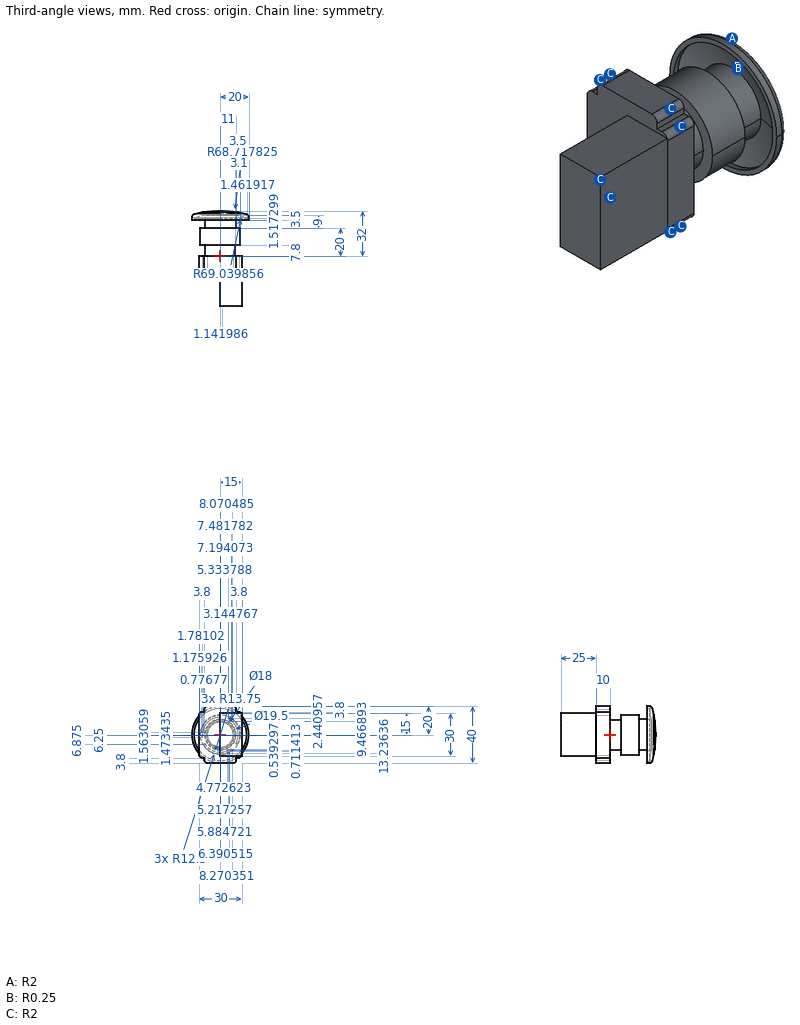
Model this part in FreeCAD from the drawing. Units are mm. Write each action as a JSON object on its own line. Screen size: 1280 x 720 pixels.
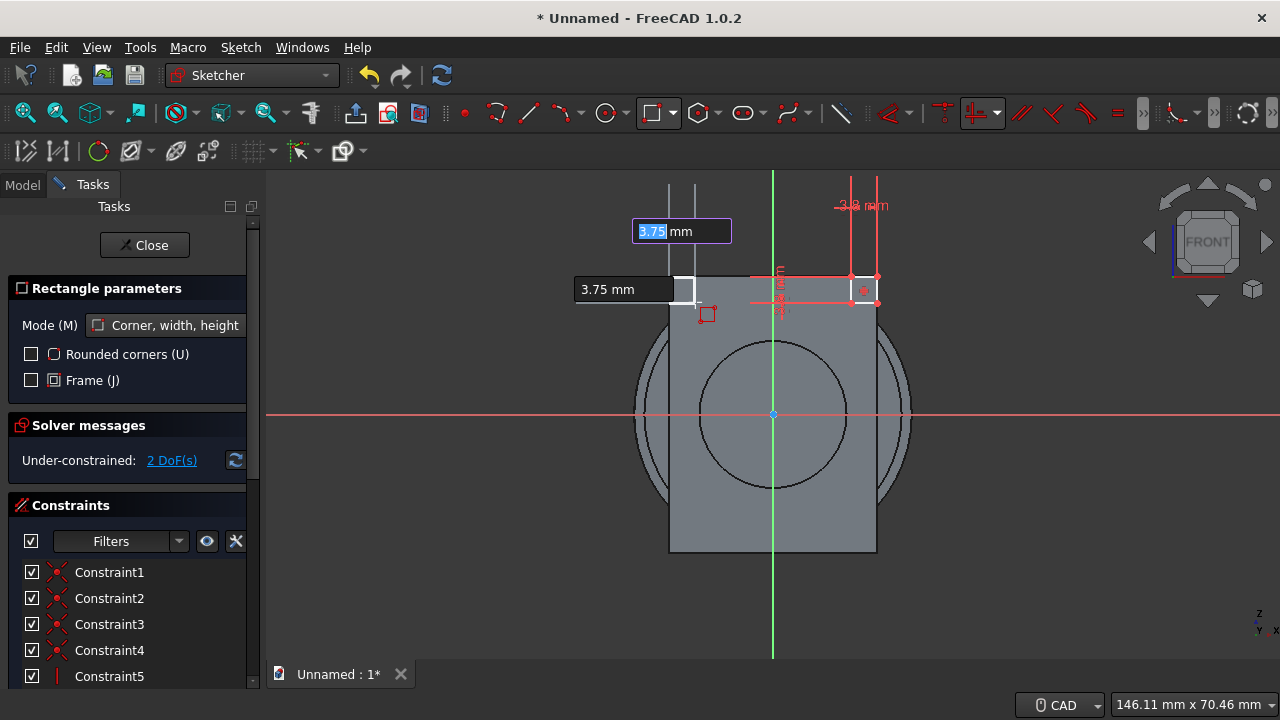
{"action": "type", "text": "3.8"}
{"action": "key", "text": "Tab"}
{"action": "type", "text": "3.8"}
{"action": "key", "text": "Return"}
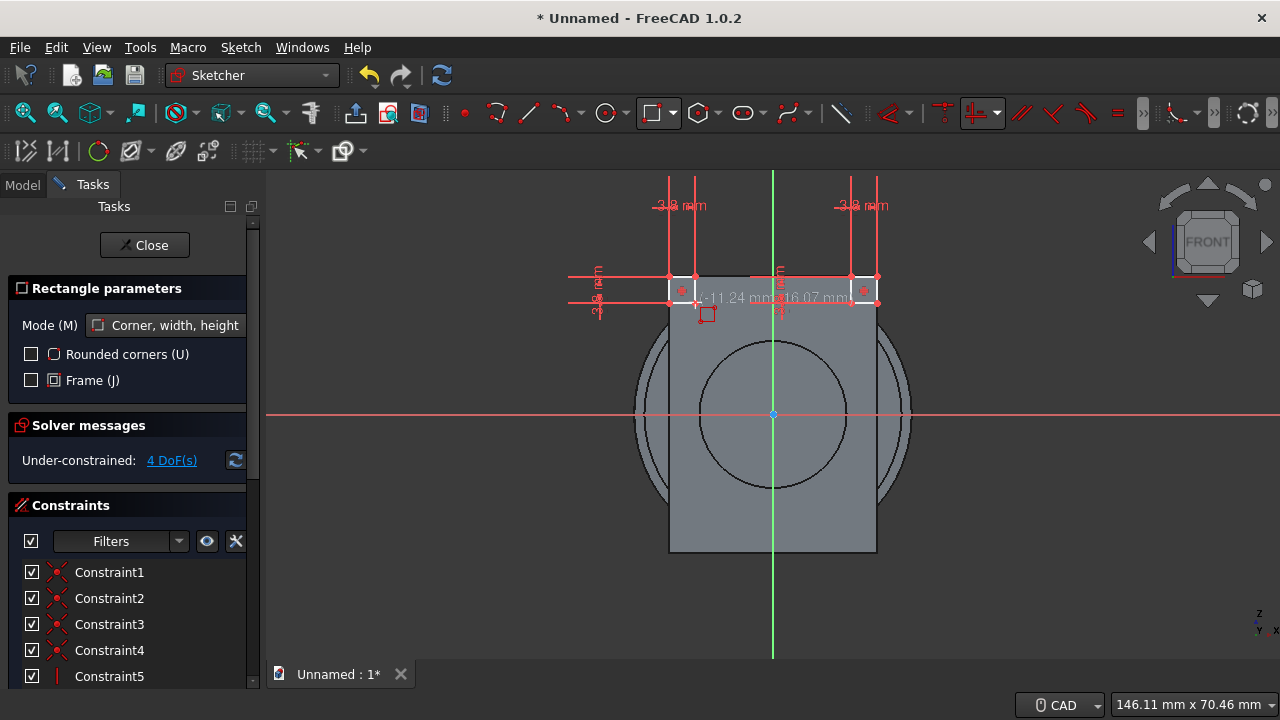
{"action": "left_click", "coordinate": [669, 527]}
{"action": "mouse_move", "coordinate": [695, 553]}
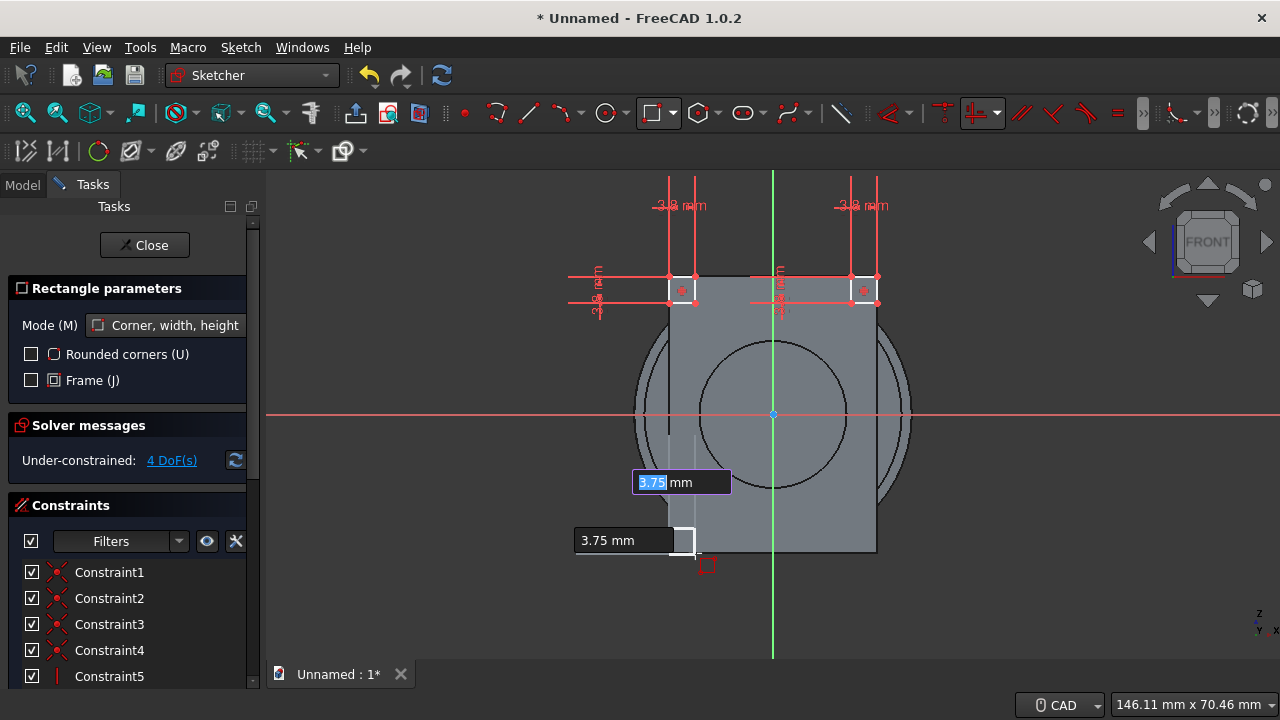
{"action": "type", "text": "3.8"}
{"action": "key", "text": "Tab"}
{"action": "type", "text": "3.8"}
{"action": "key", "text": "Return"}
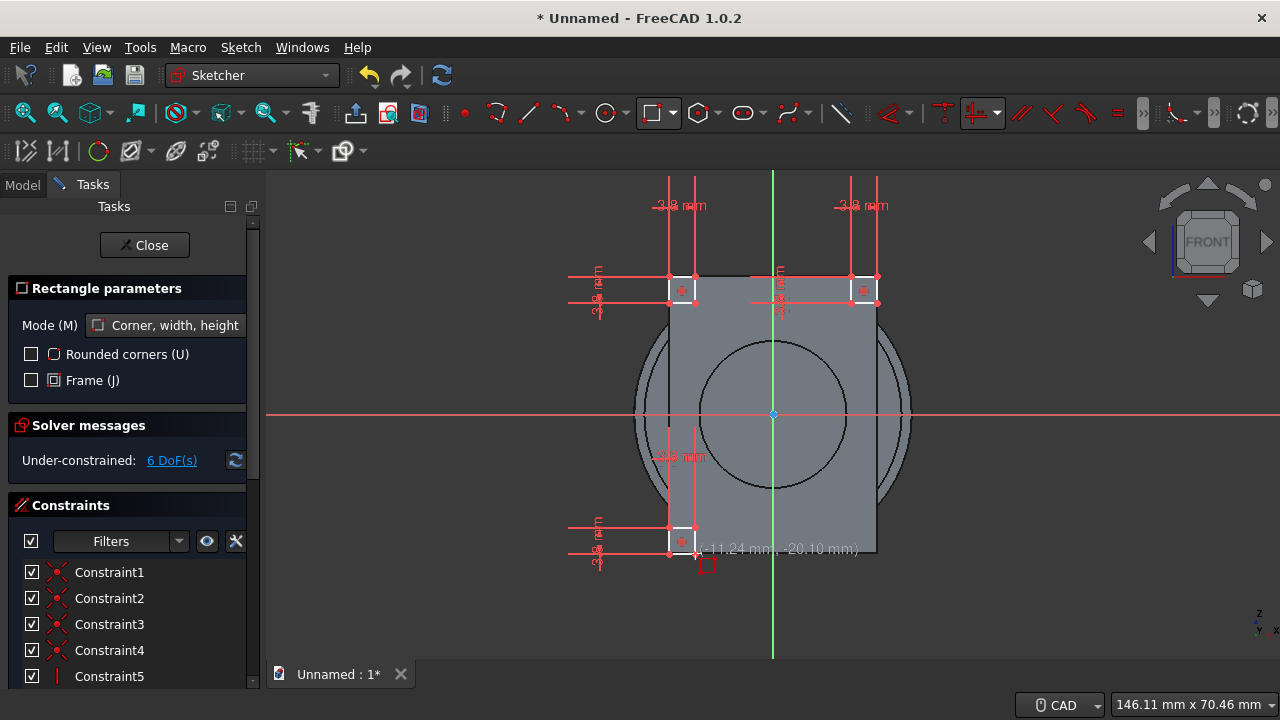
{"action": "left_click", "coordinate": [851, 527]}
{"action": "mouse_move", "coordinate": [877, 553]}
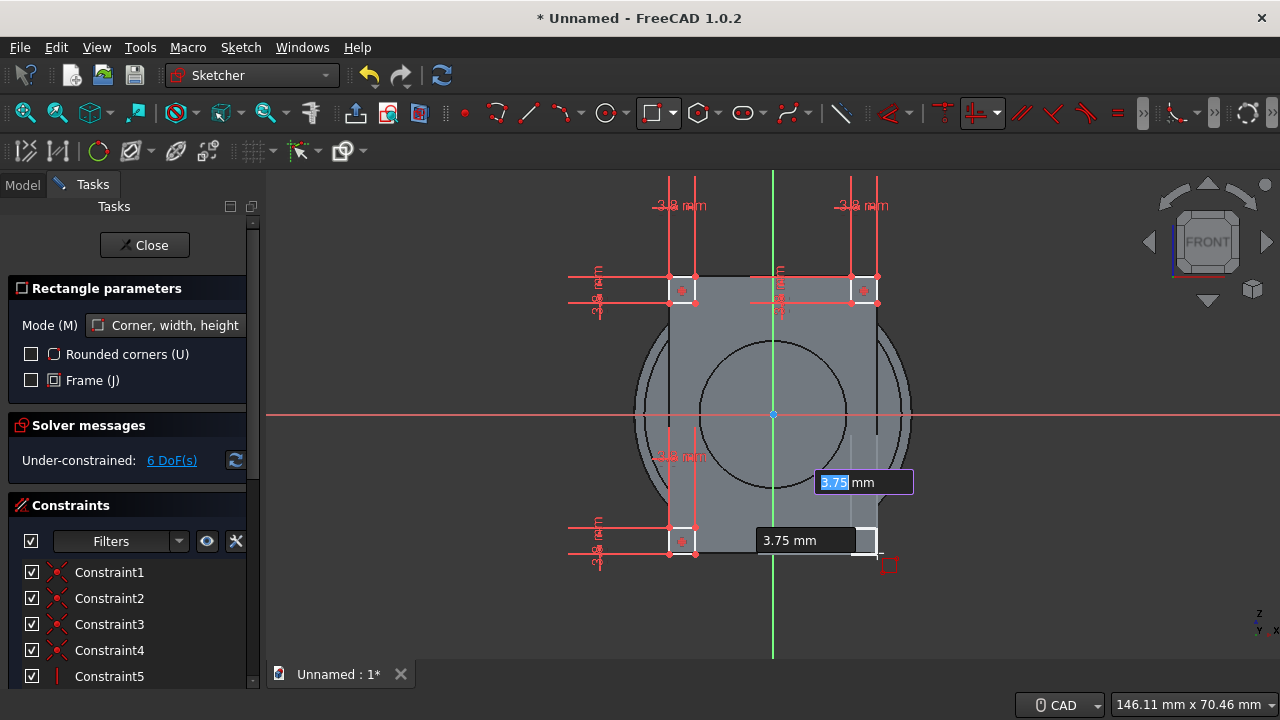
{"action": "type", "text": "3.8"}
{"action": "key", "text": "Tab"}
{"action": "type", "text": "3.8"}
{"action": "key", "text": "Return"}
{"action": "key", "text": "Escape"}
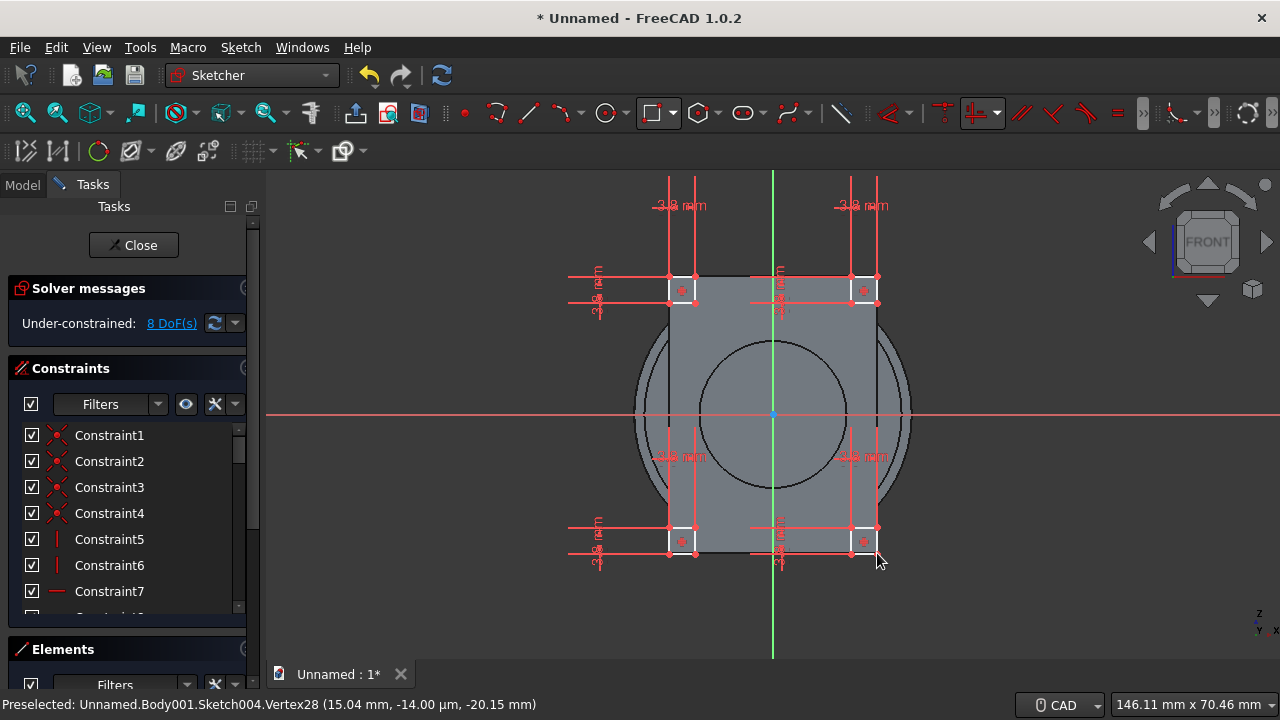
{"action": "left_click", "coordinate": [877, 277]}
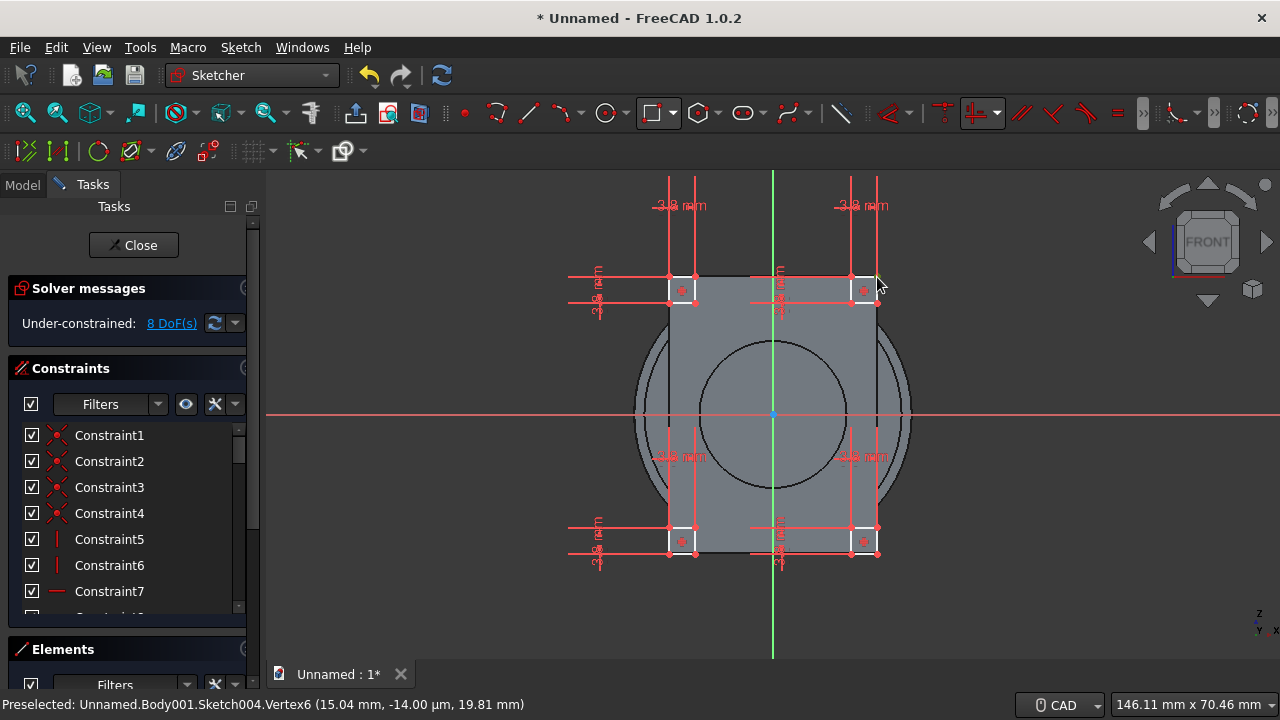
{"action": "left_click", "coordinate": [669, 277]}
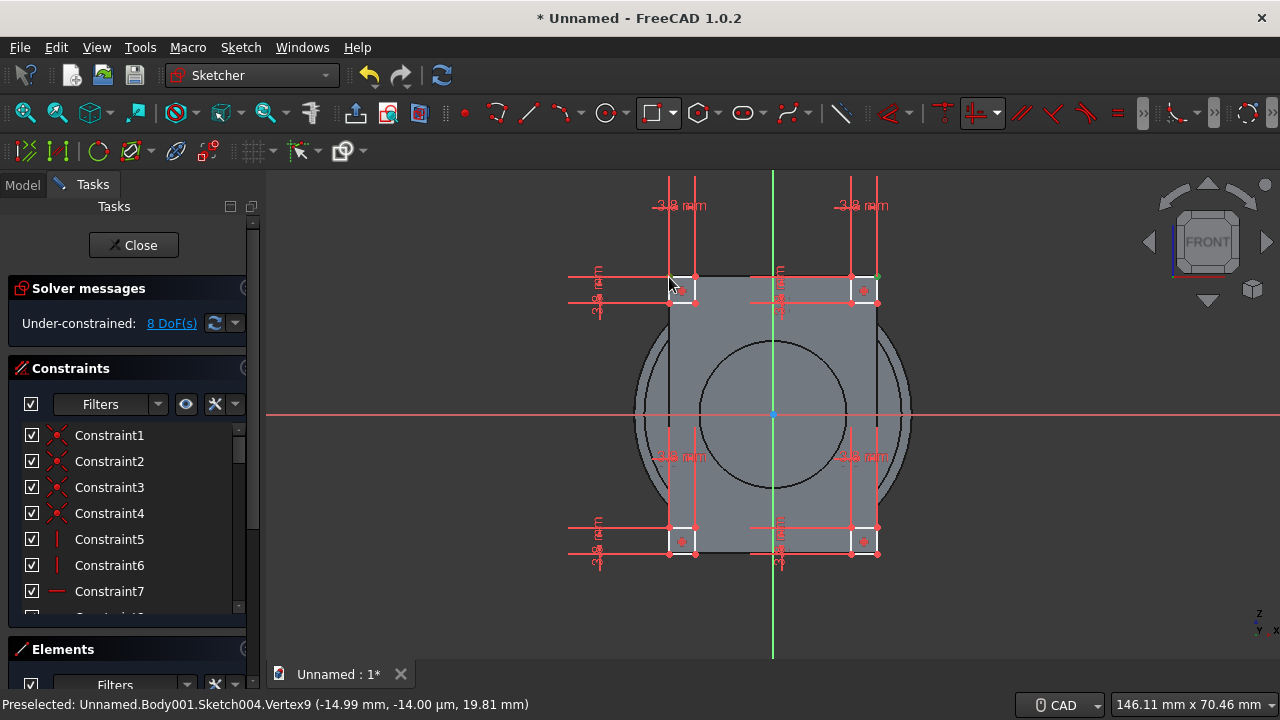
{"action": "left_click", "coordinate": [773, 600]}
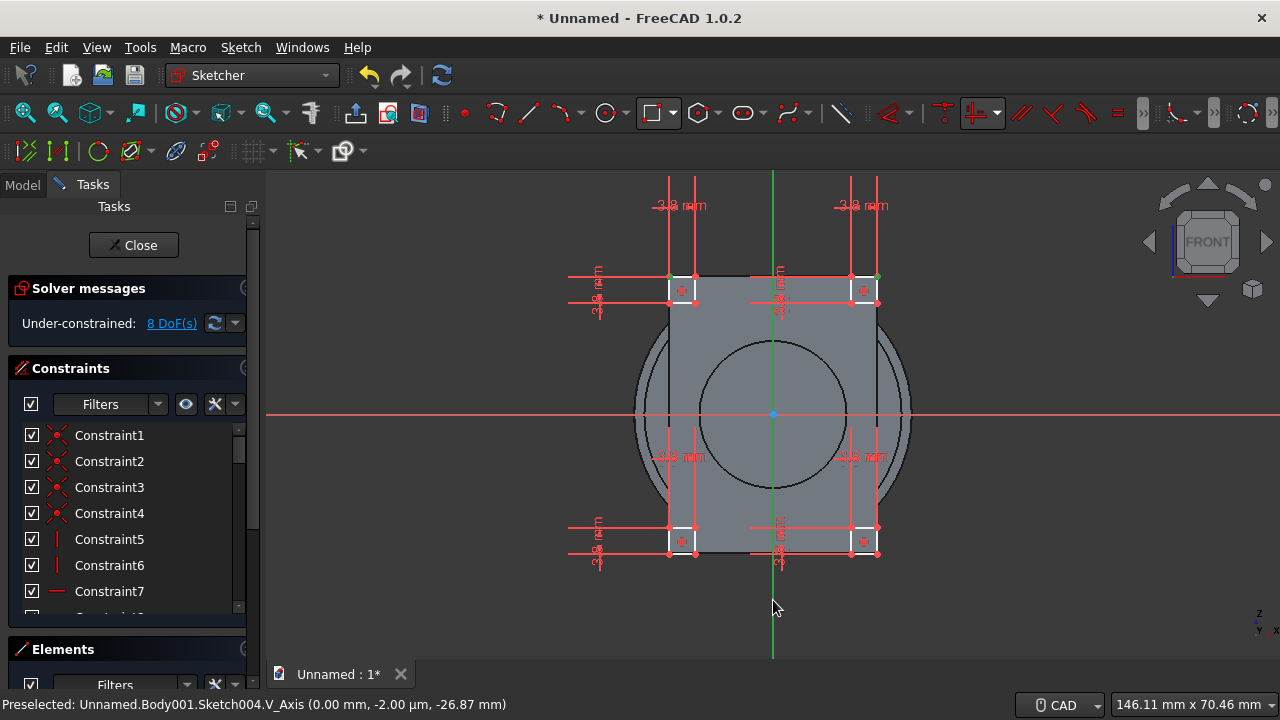
{"action": "key", "text": "s"}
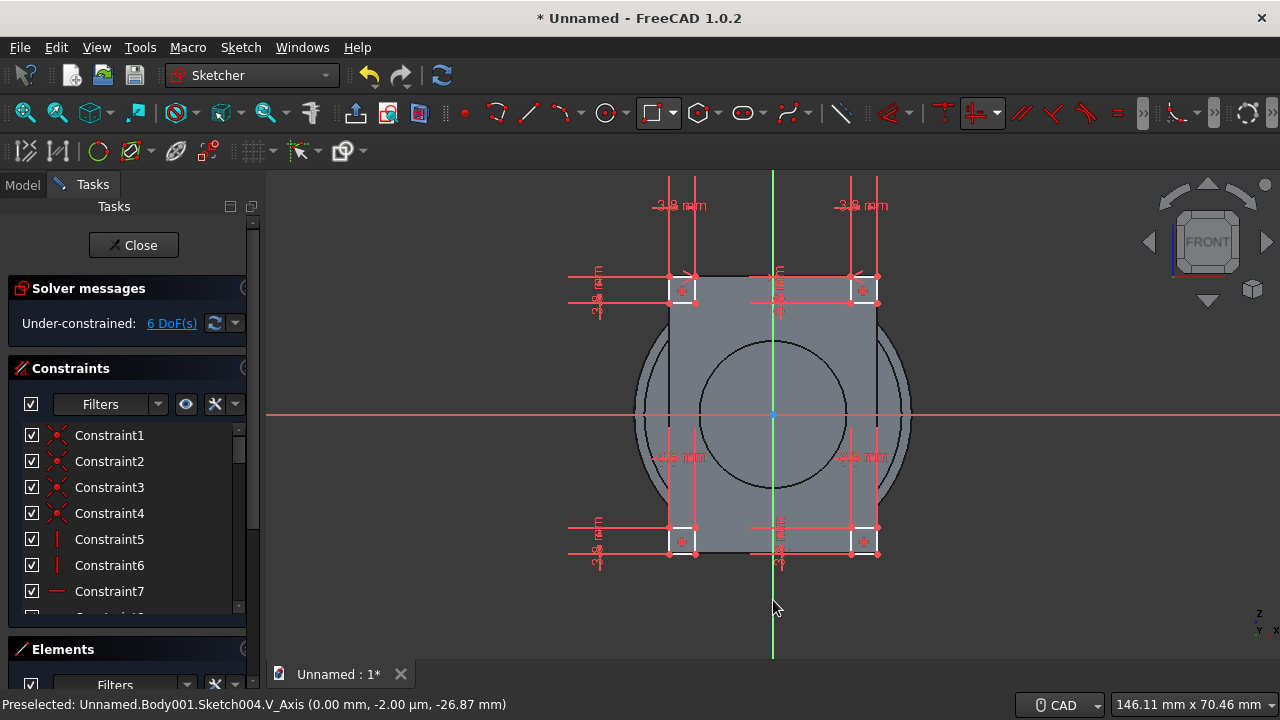
{"action": "left_click", "coordinate": [669, 303]}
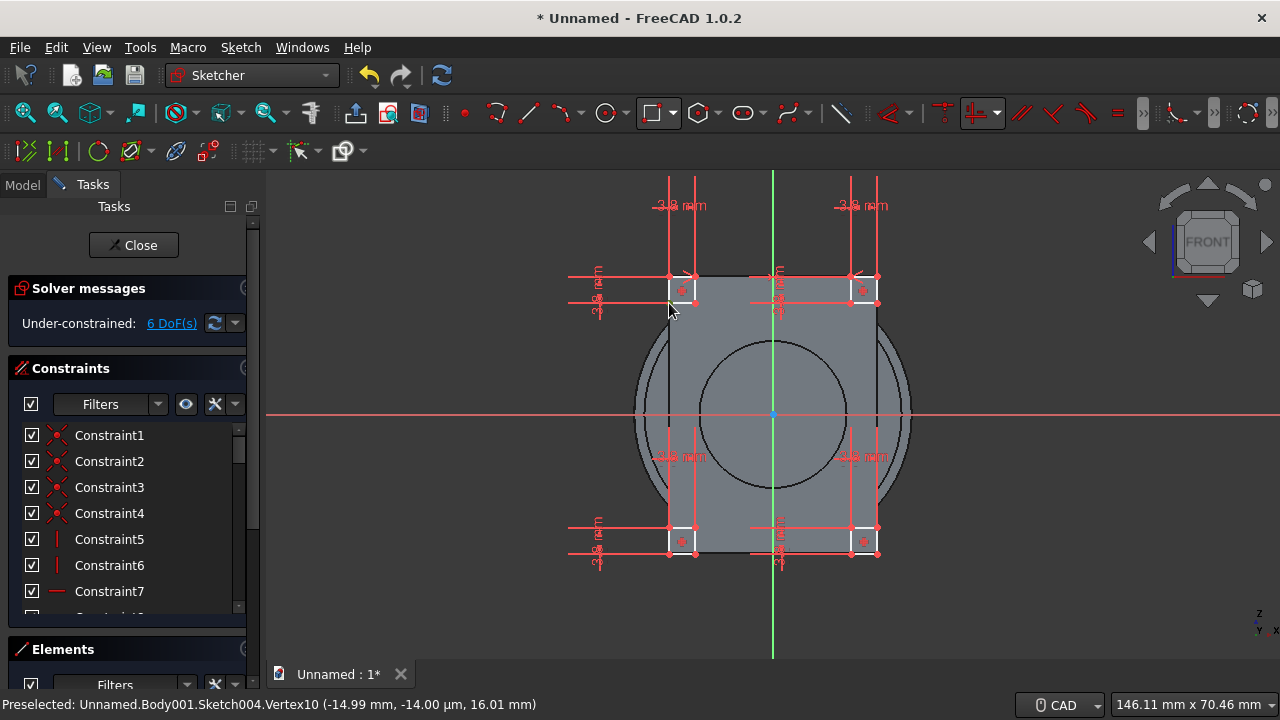
{"action": "left_click", "coordinate": [669, 528]}